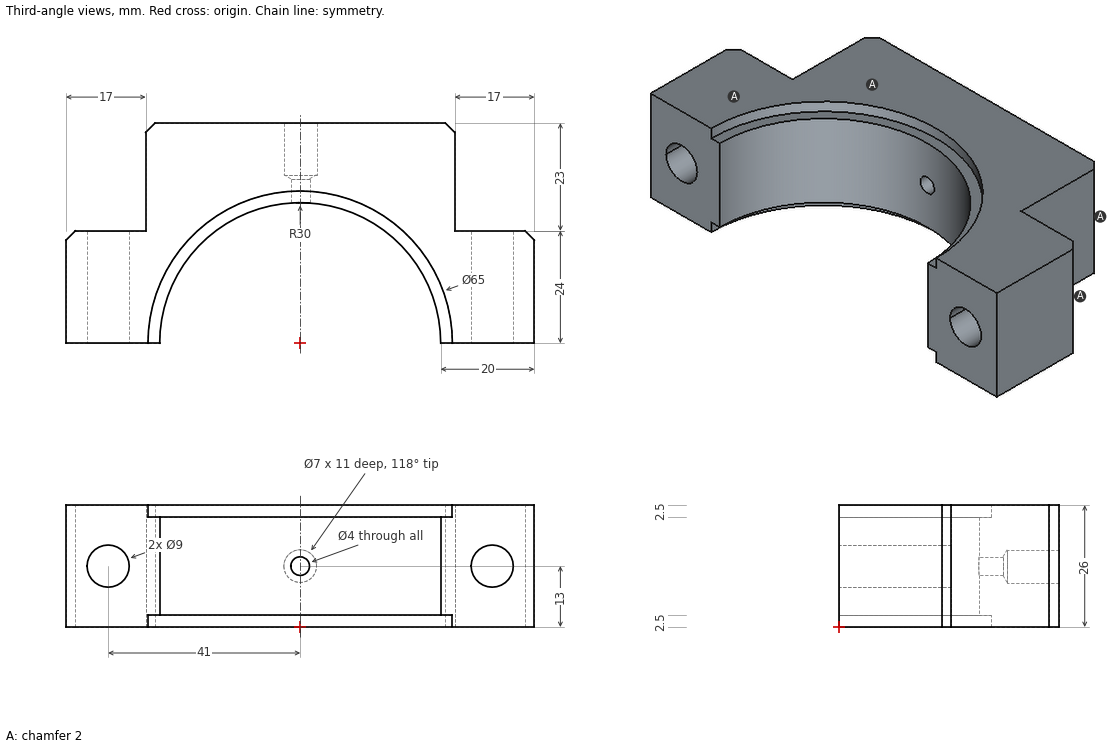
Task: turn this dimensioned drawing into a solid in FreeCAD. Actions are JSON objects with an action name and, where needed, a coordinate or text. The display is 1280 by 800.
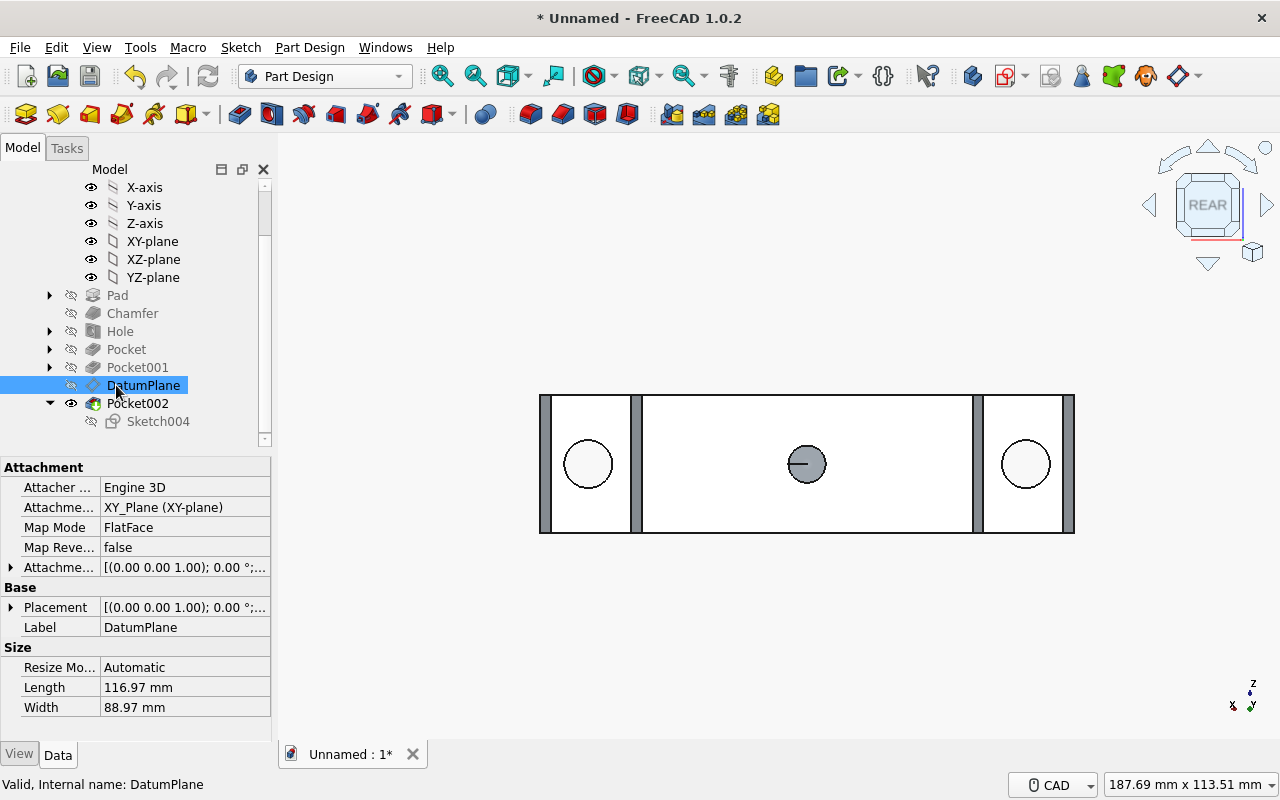
{"action": "left_click", "coordinate": [713, 463]}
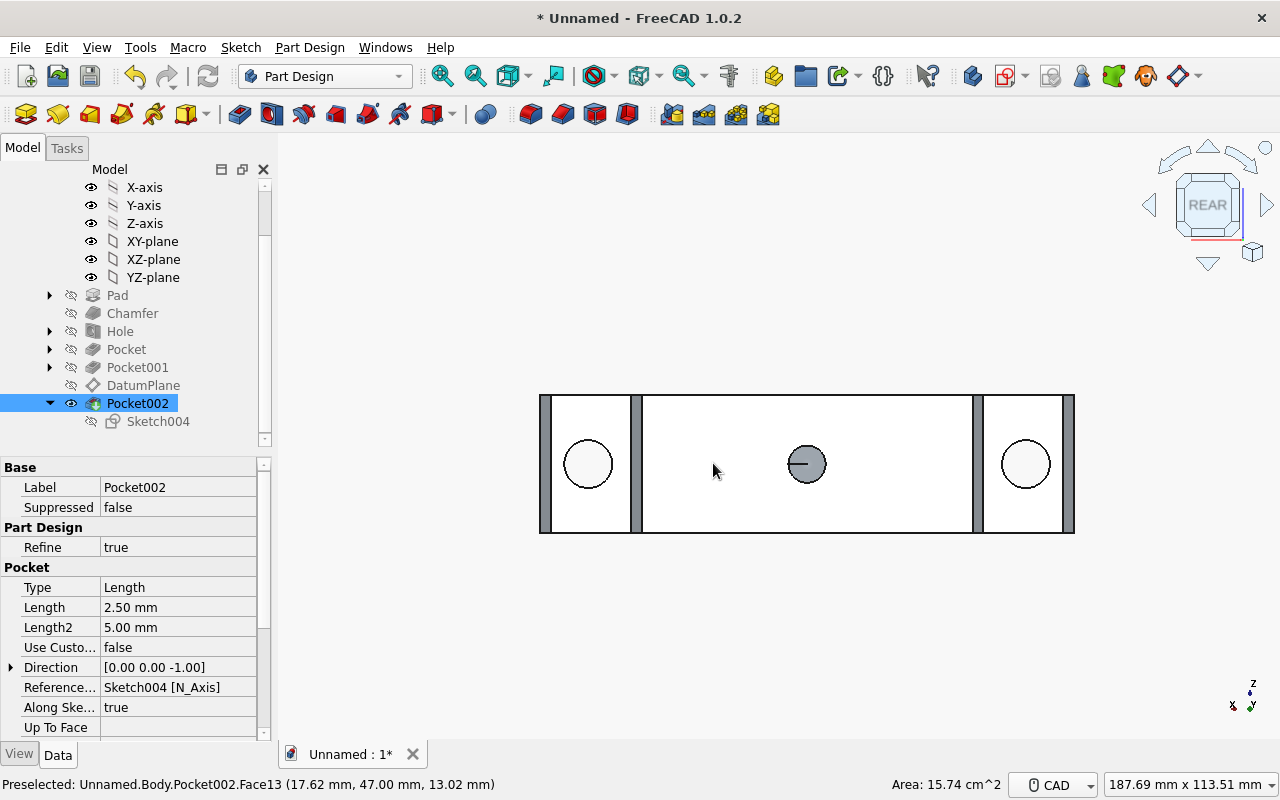
{"action": "left_click", "coordinate": [1006, 76]}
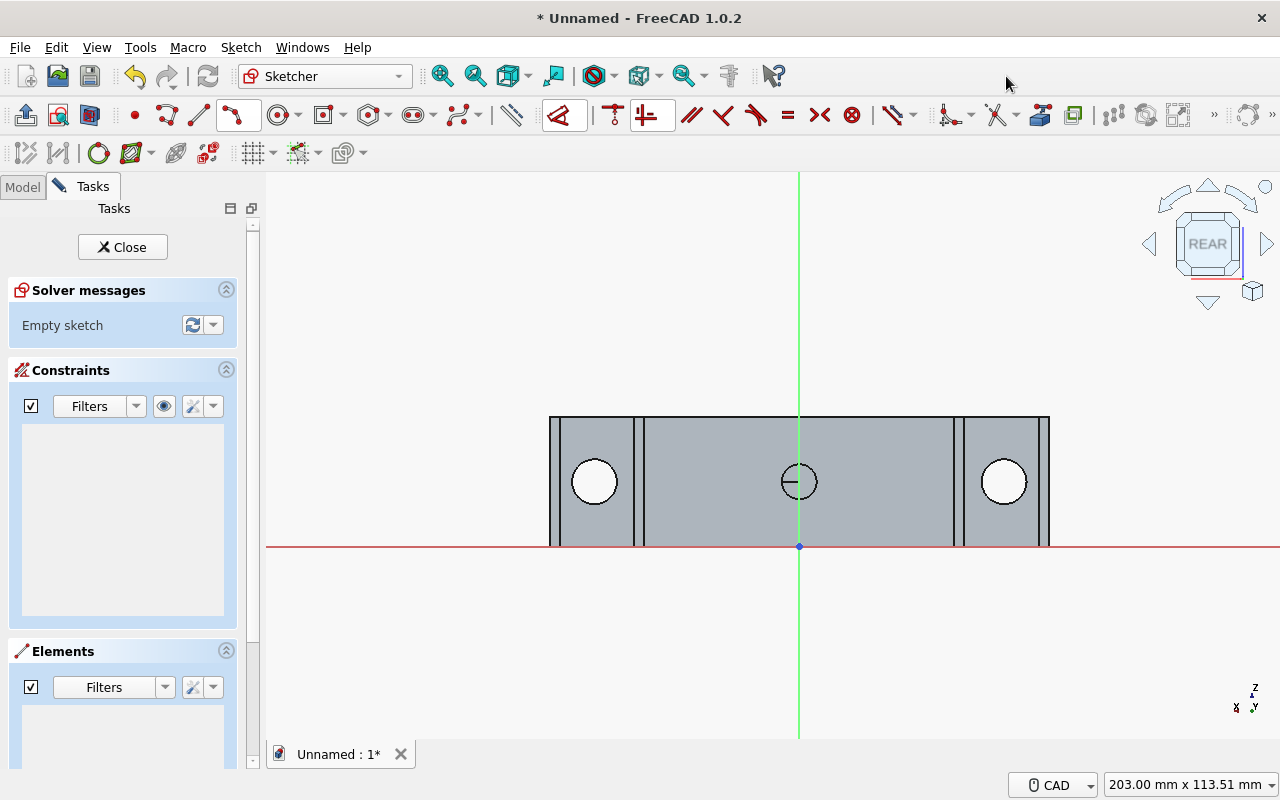
{"action": "scroll", "coordinate": [805, 483], "scroll_direction": "up", "scroll_amount": 14}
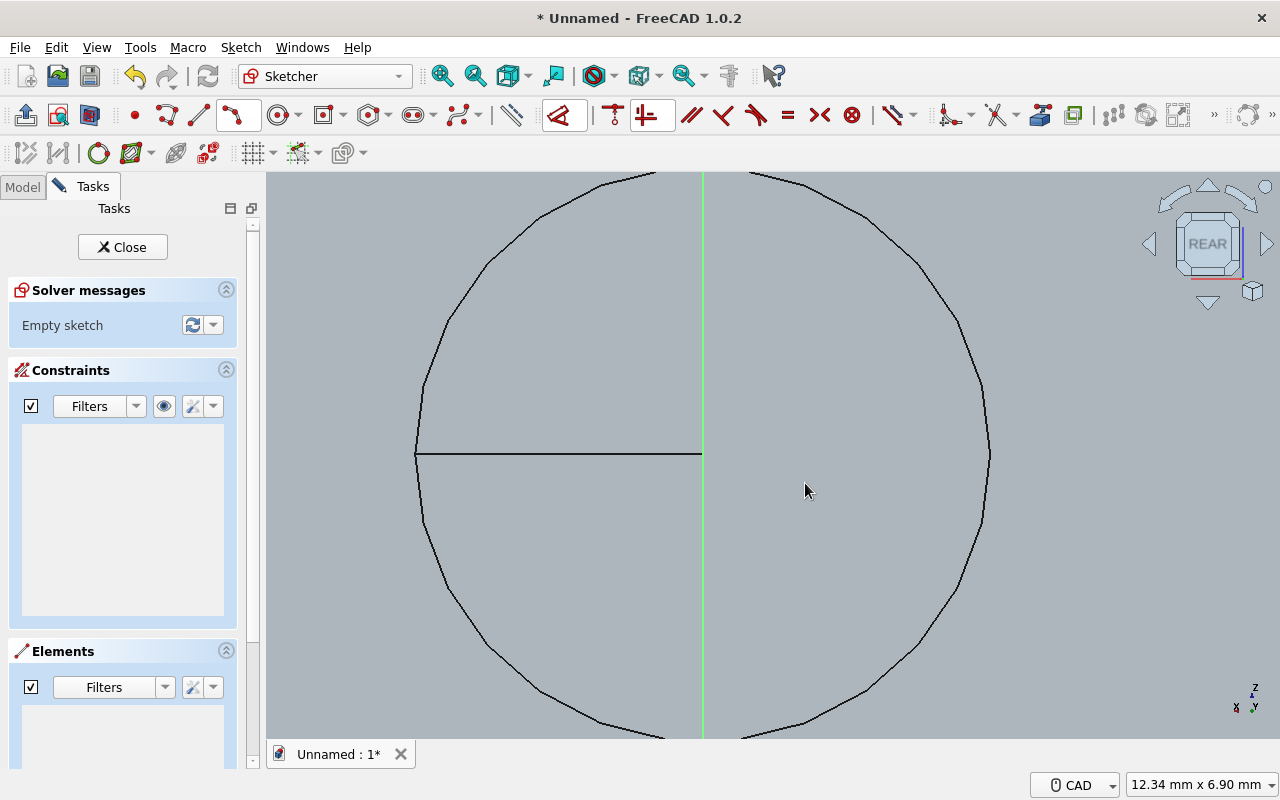
{"action": "left_click", "coordinate": [278, 116]}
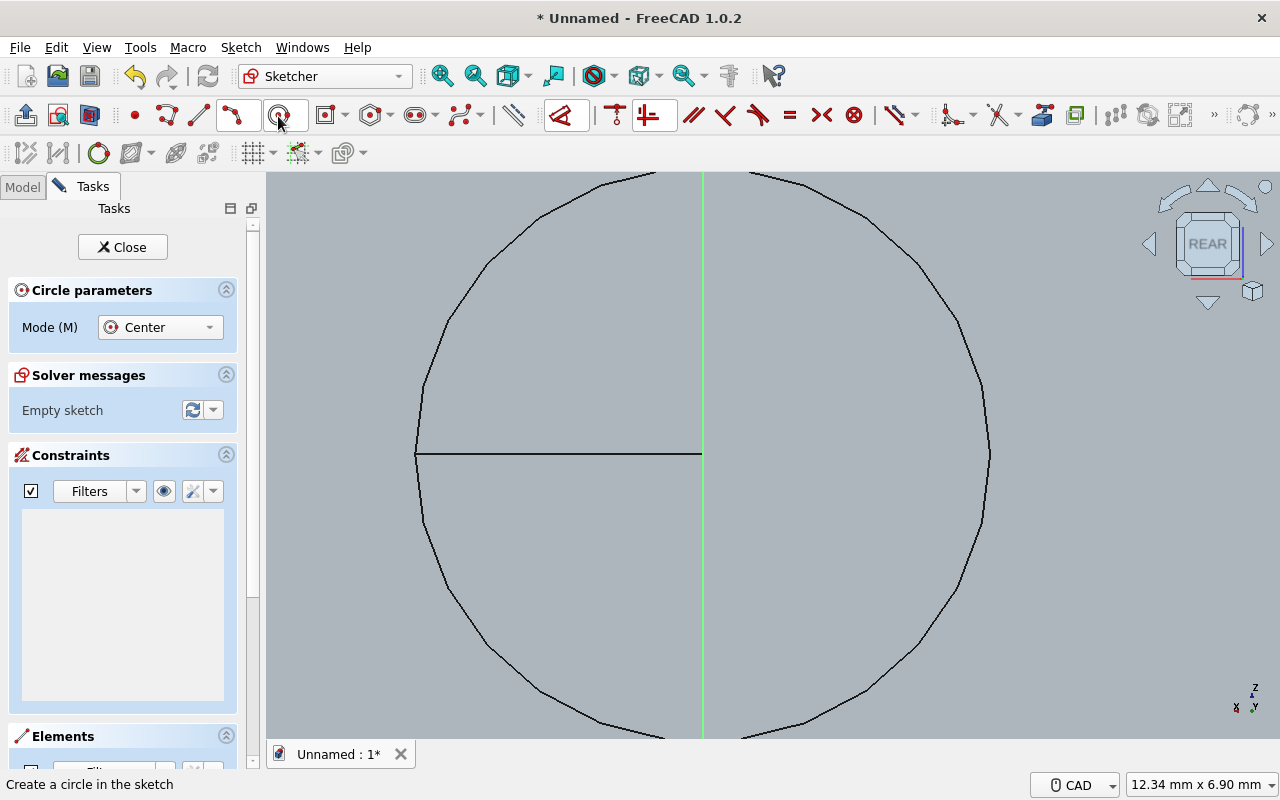
{"action": "left_click", "coordinate": [703, 454]}
{"action": "left_click", "coordinate": [819, 338]}
{"action": "key", "text": "Escape"}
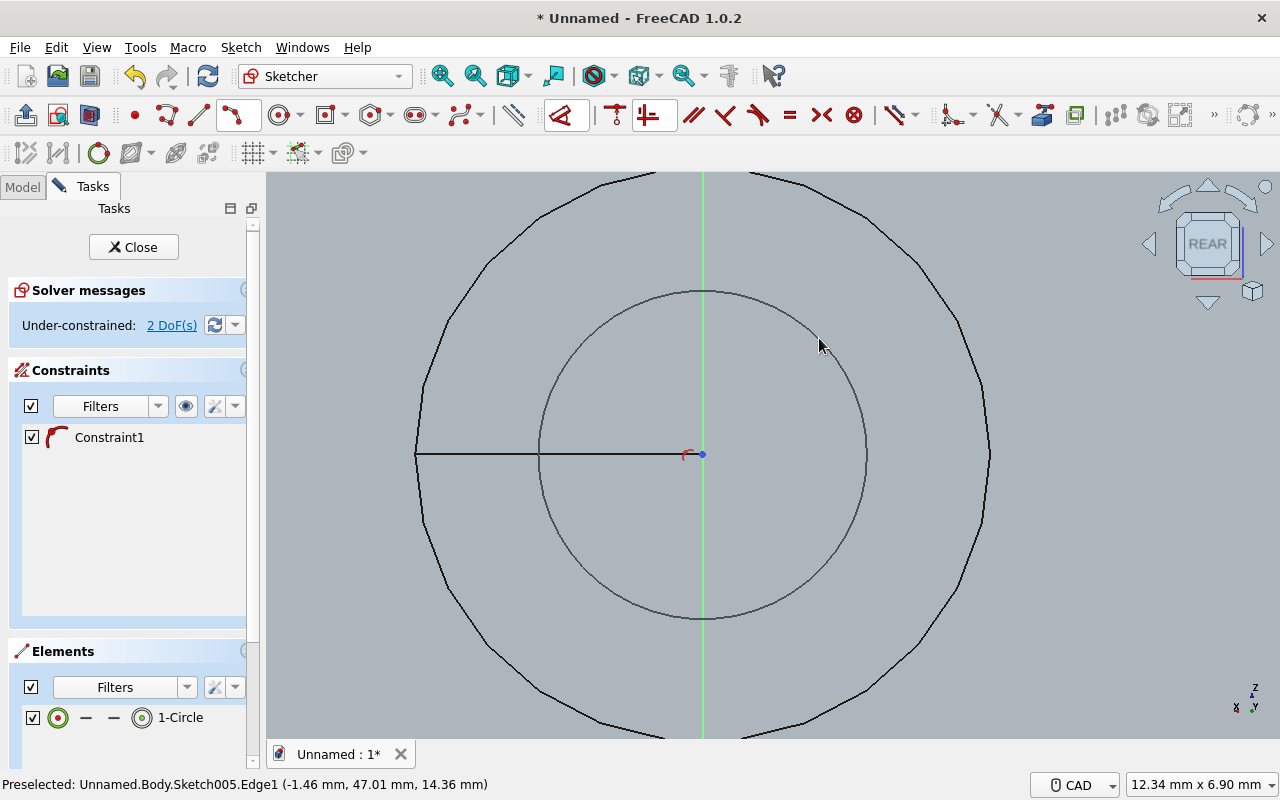
{"action": "left_click", "coordinate": [818, 338]}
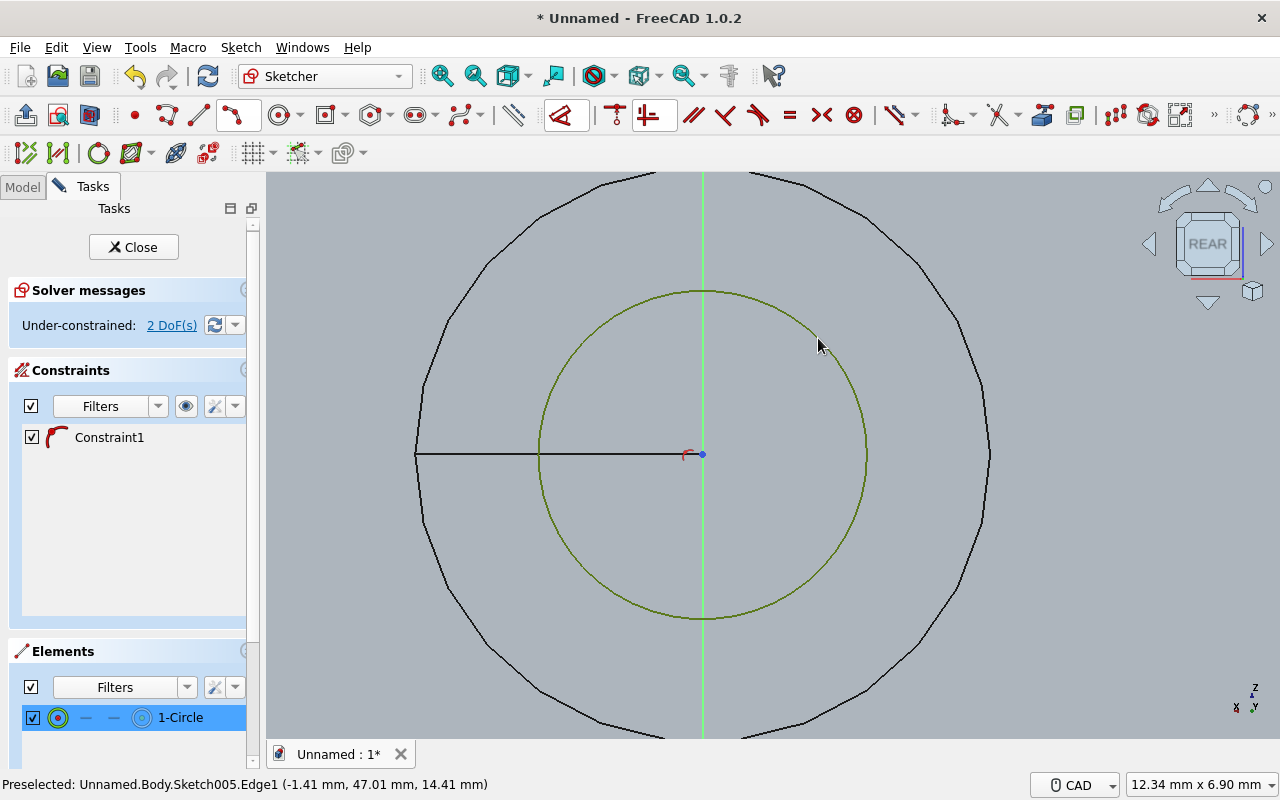
{"action": "key", "text": "k o"}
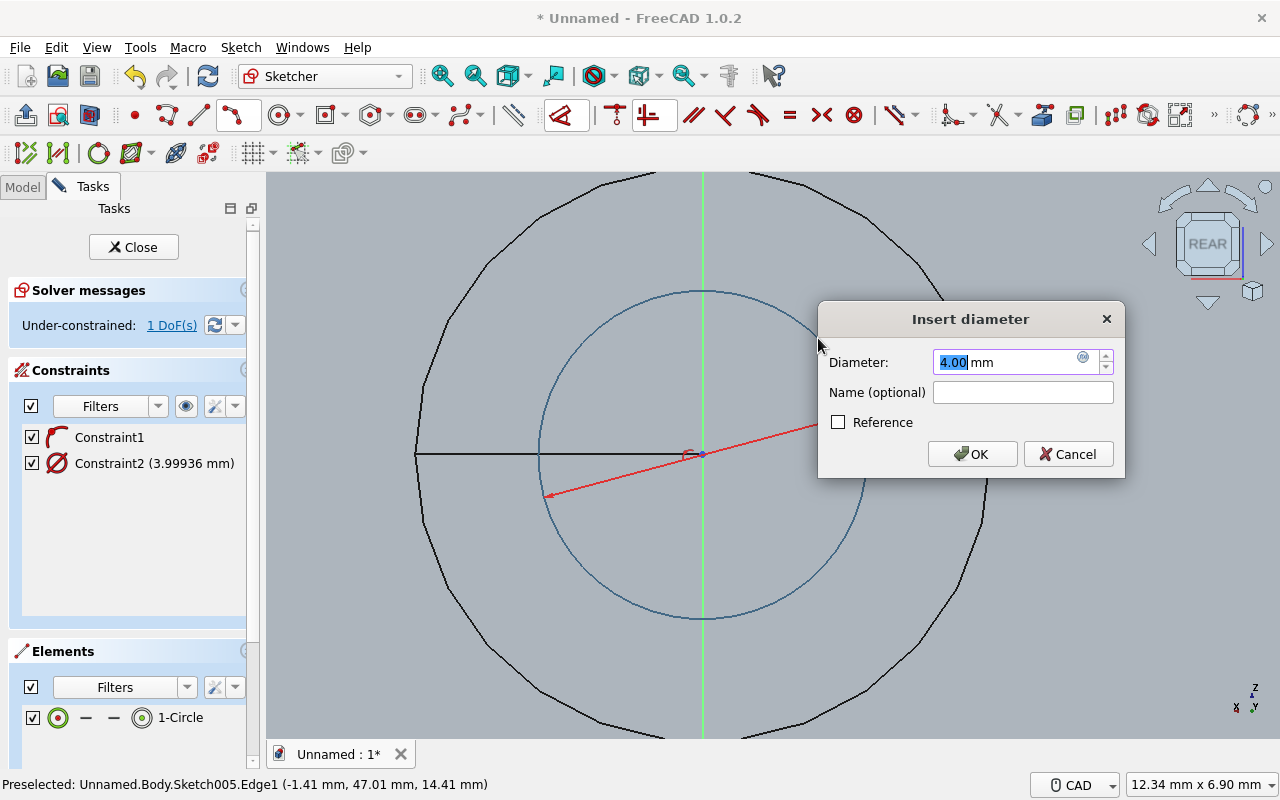
{"action": "type", "text": "4"}
{"action": "key", "text": "Return"}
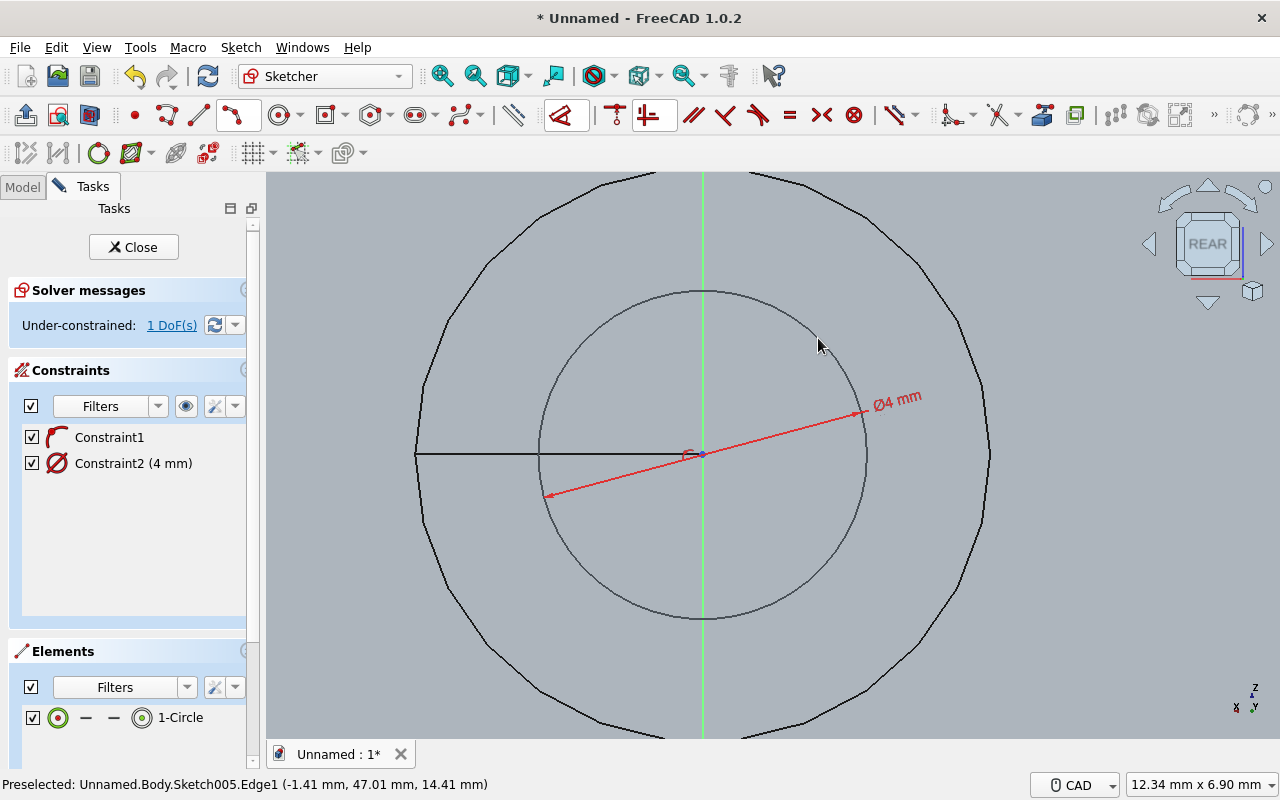
{"action": "left_click", "coordinate": [703, 455]}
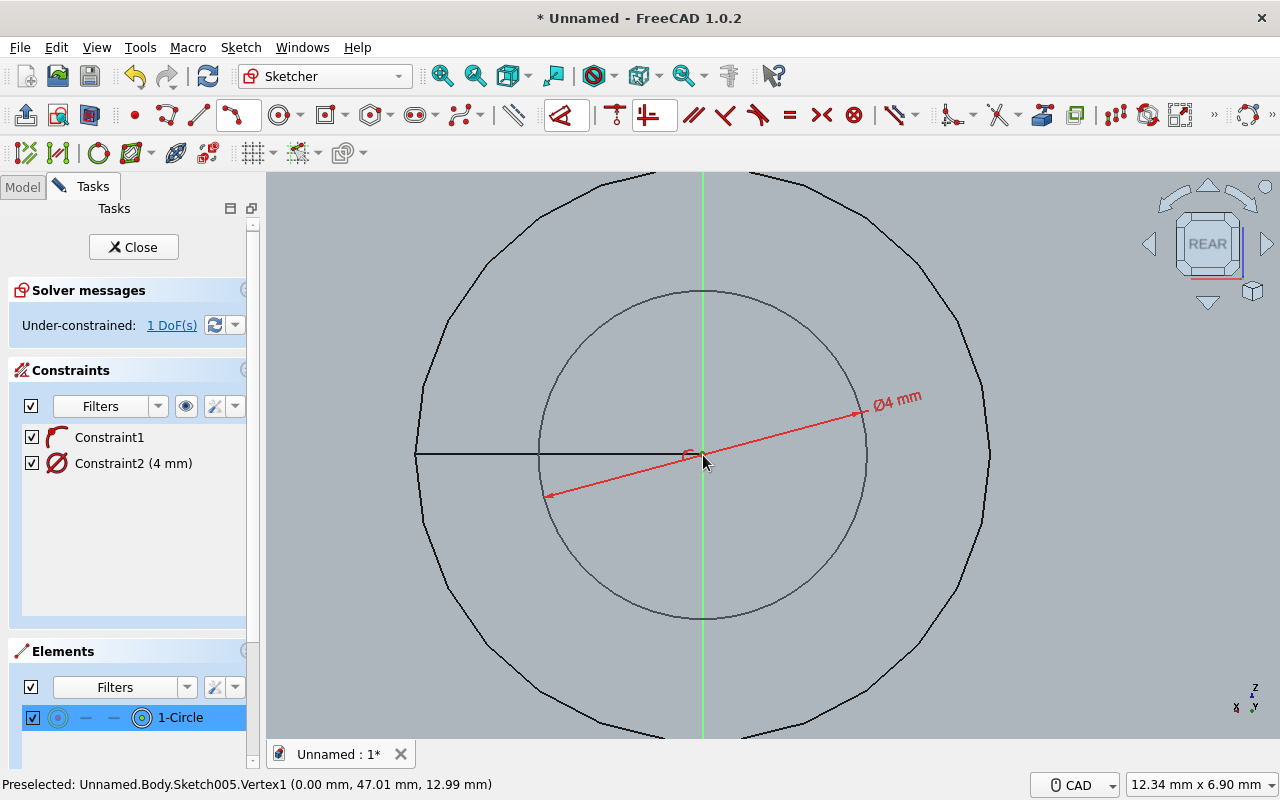
{"action": "key", "text": "i"}